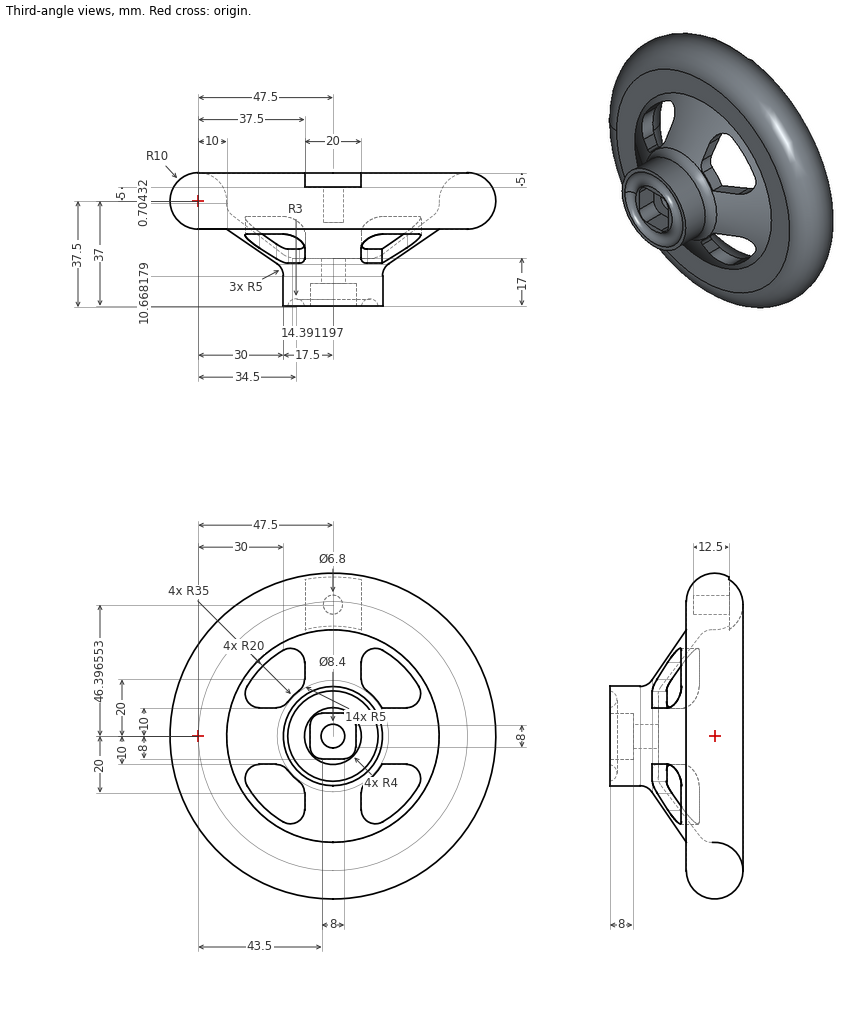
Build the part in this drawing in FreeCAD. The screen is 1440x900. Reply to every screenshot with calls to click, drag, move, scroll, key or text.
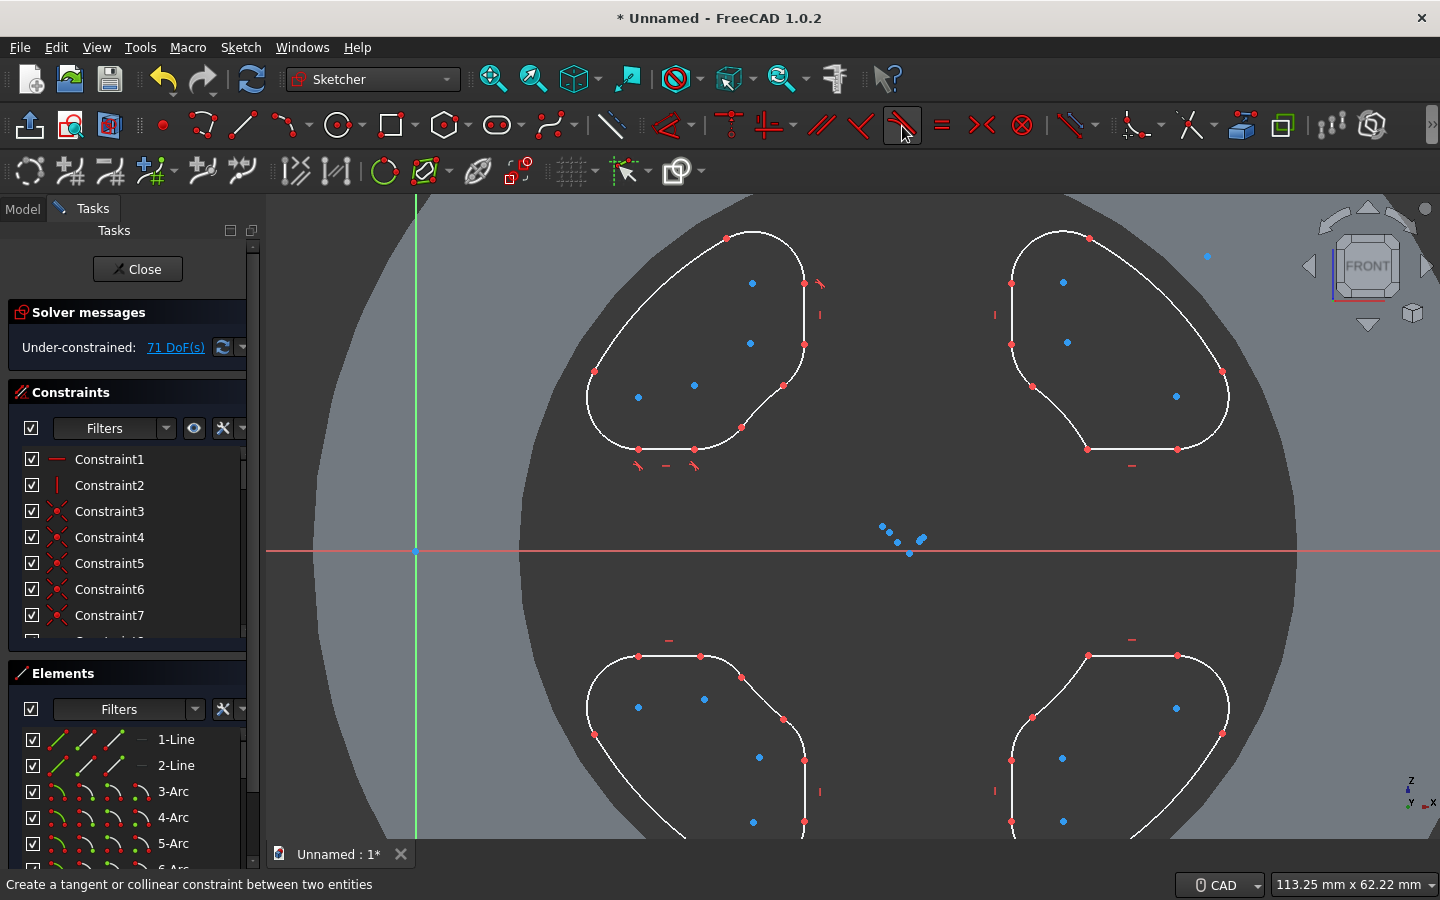
click(804, 302)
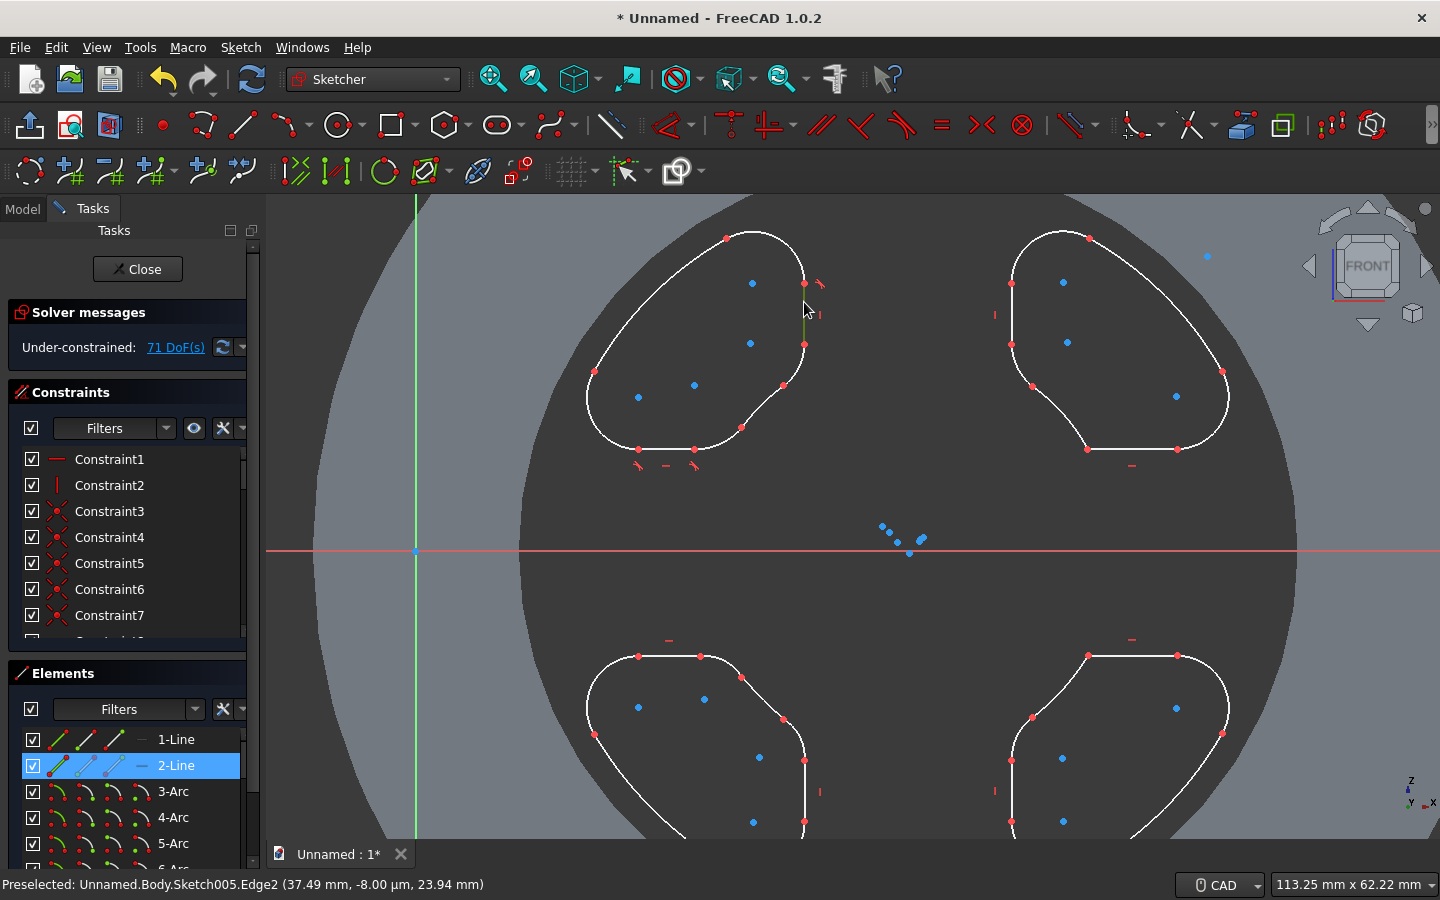
click(794, 376)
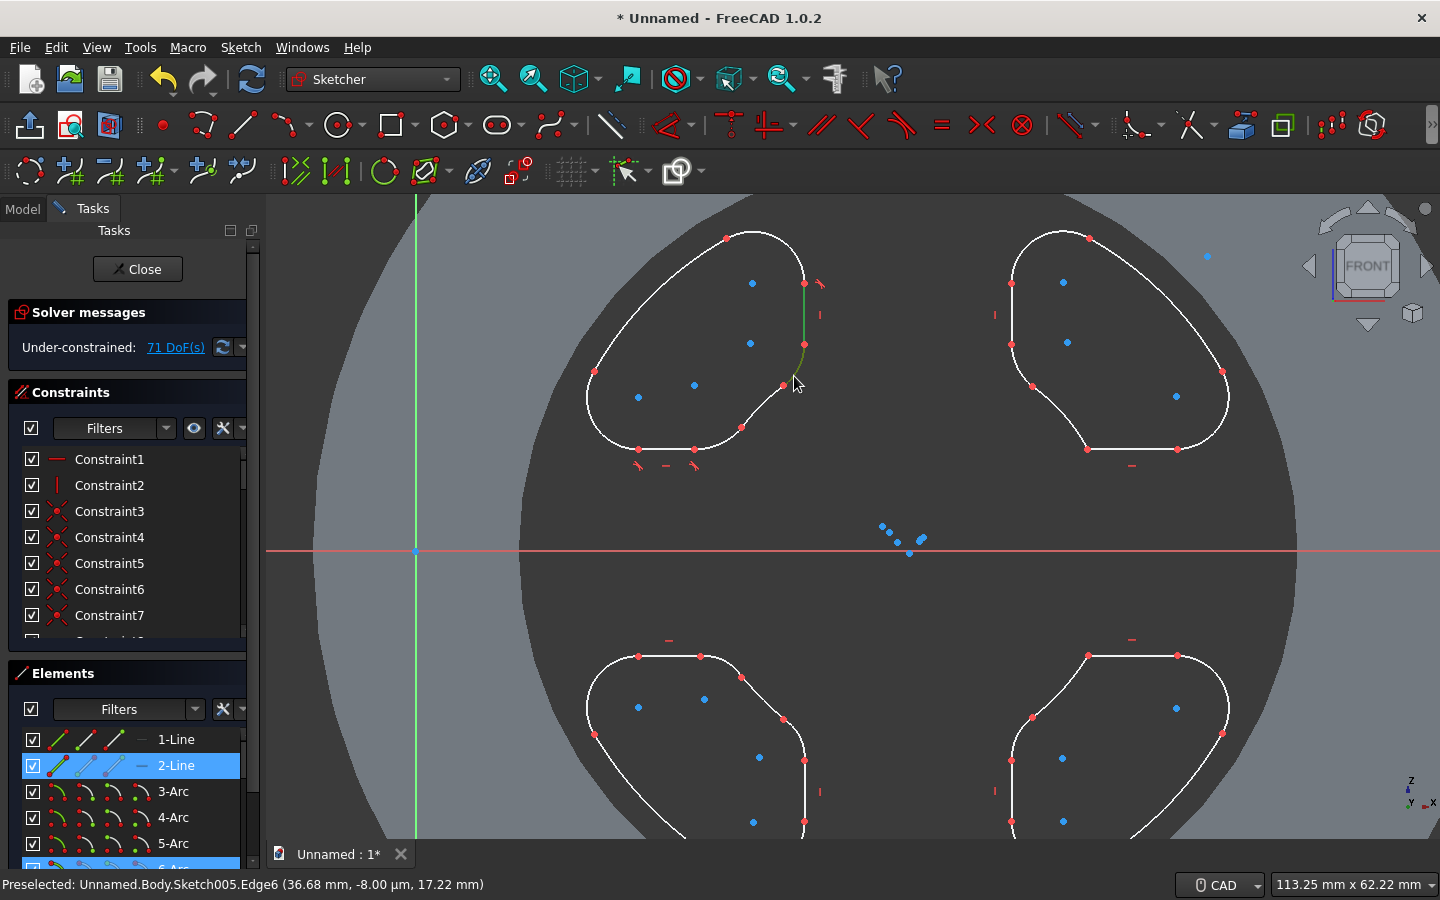
click(902, 126)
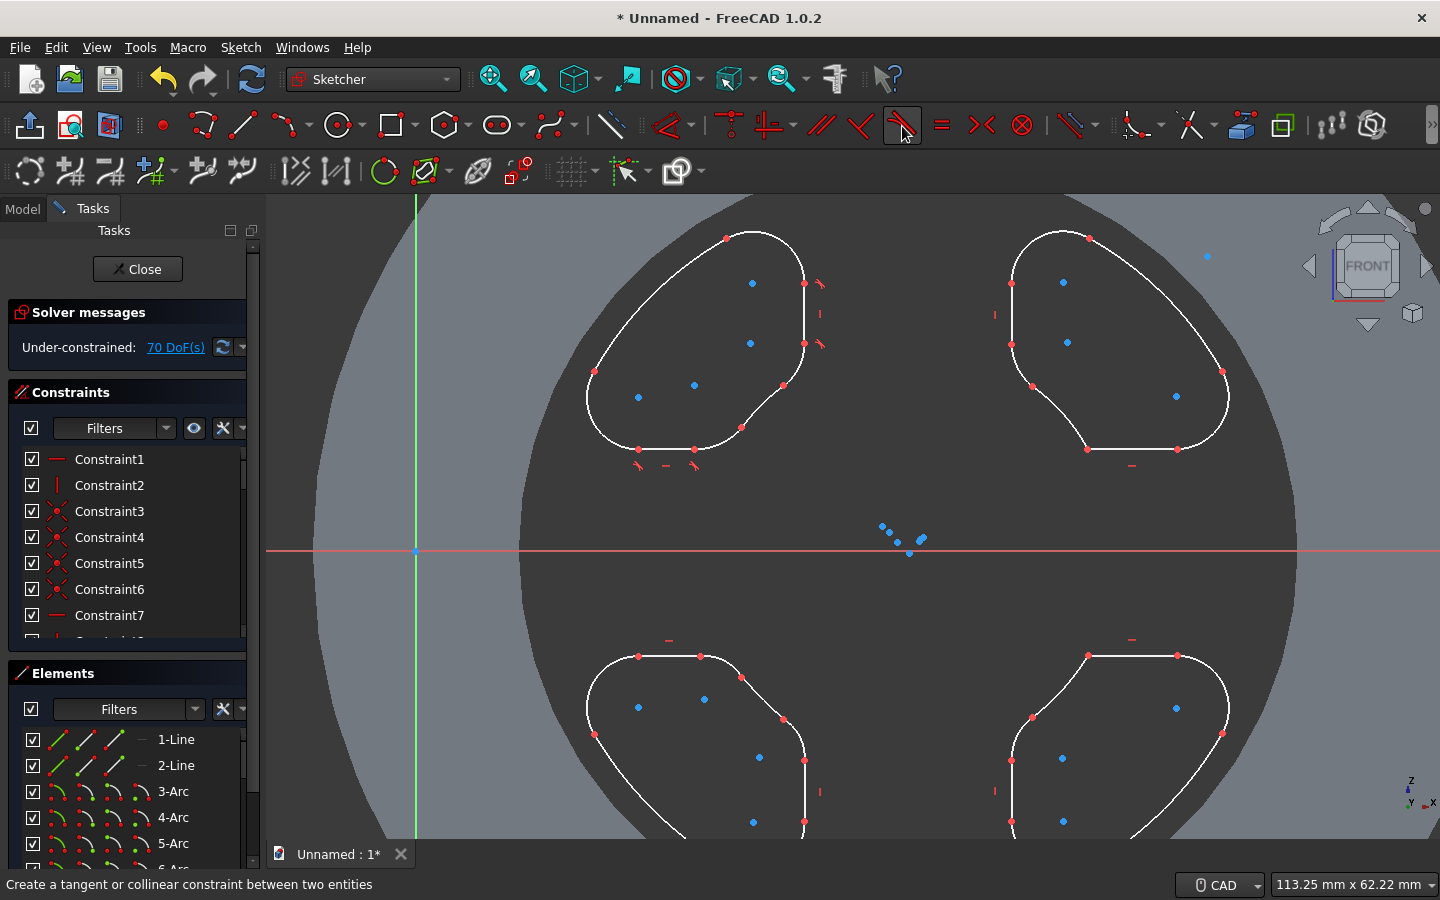
click(587, 403)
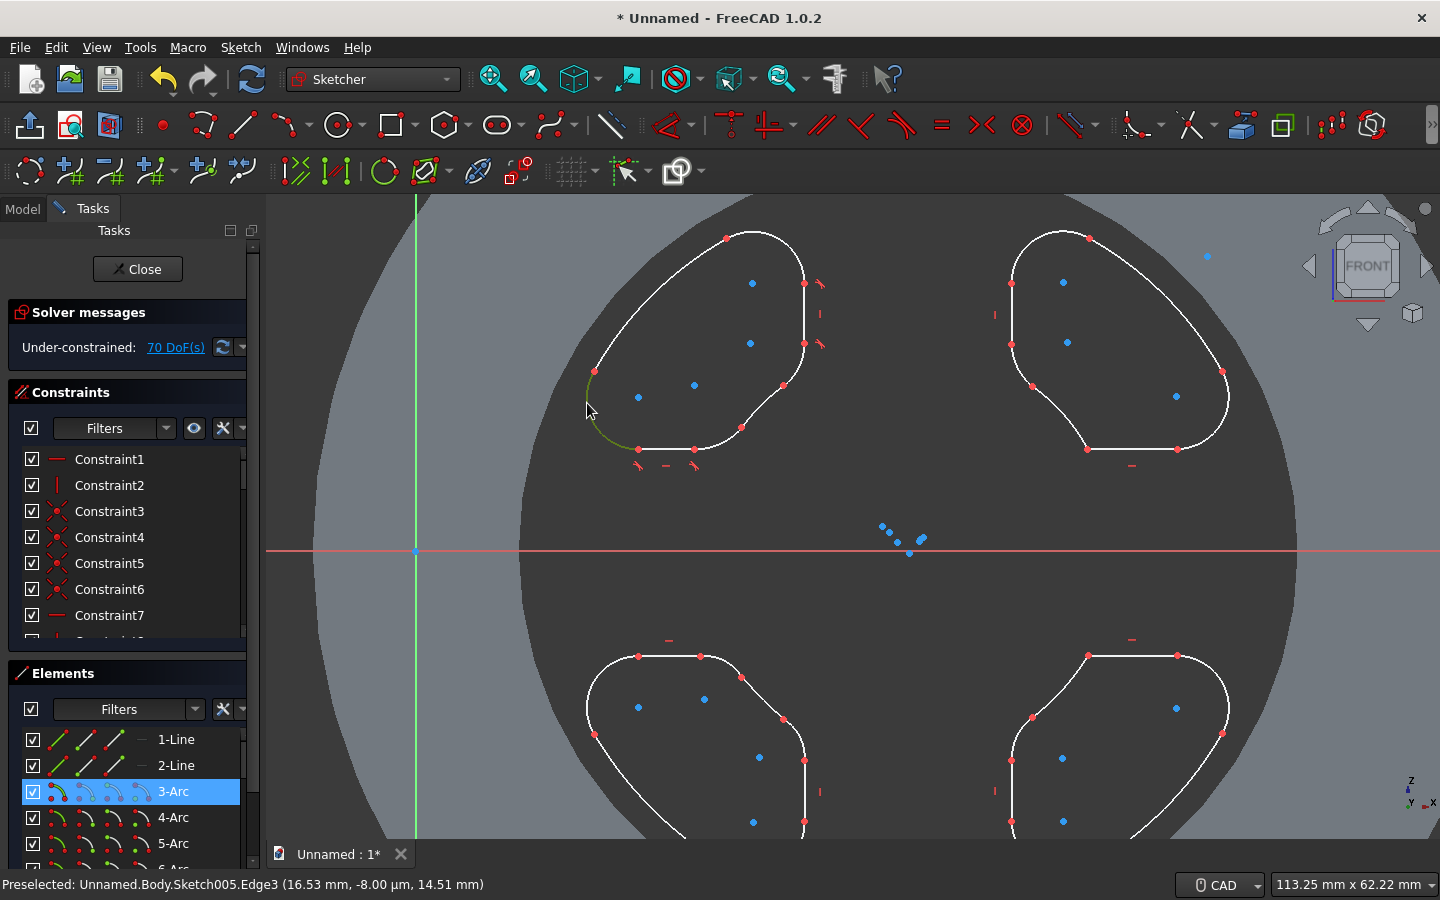
click(680, 271)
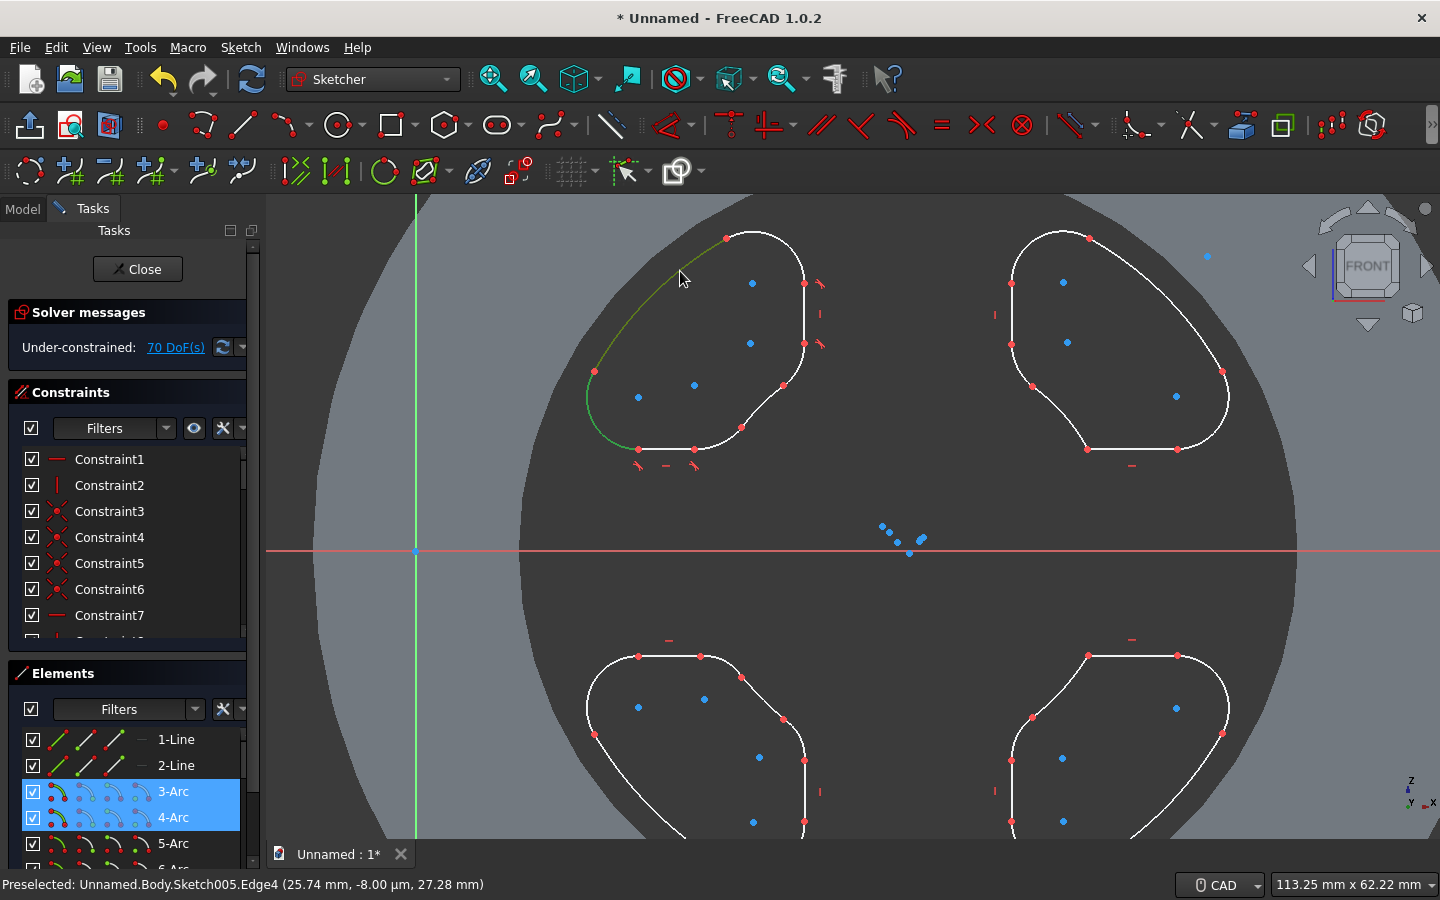
click(902, 126)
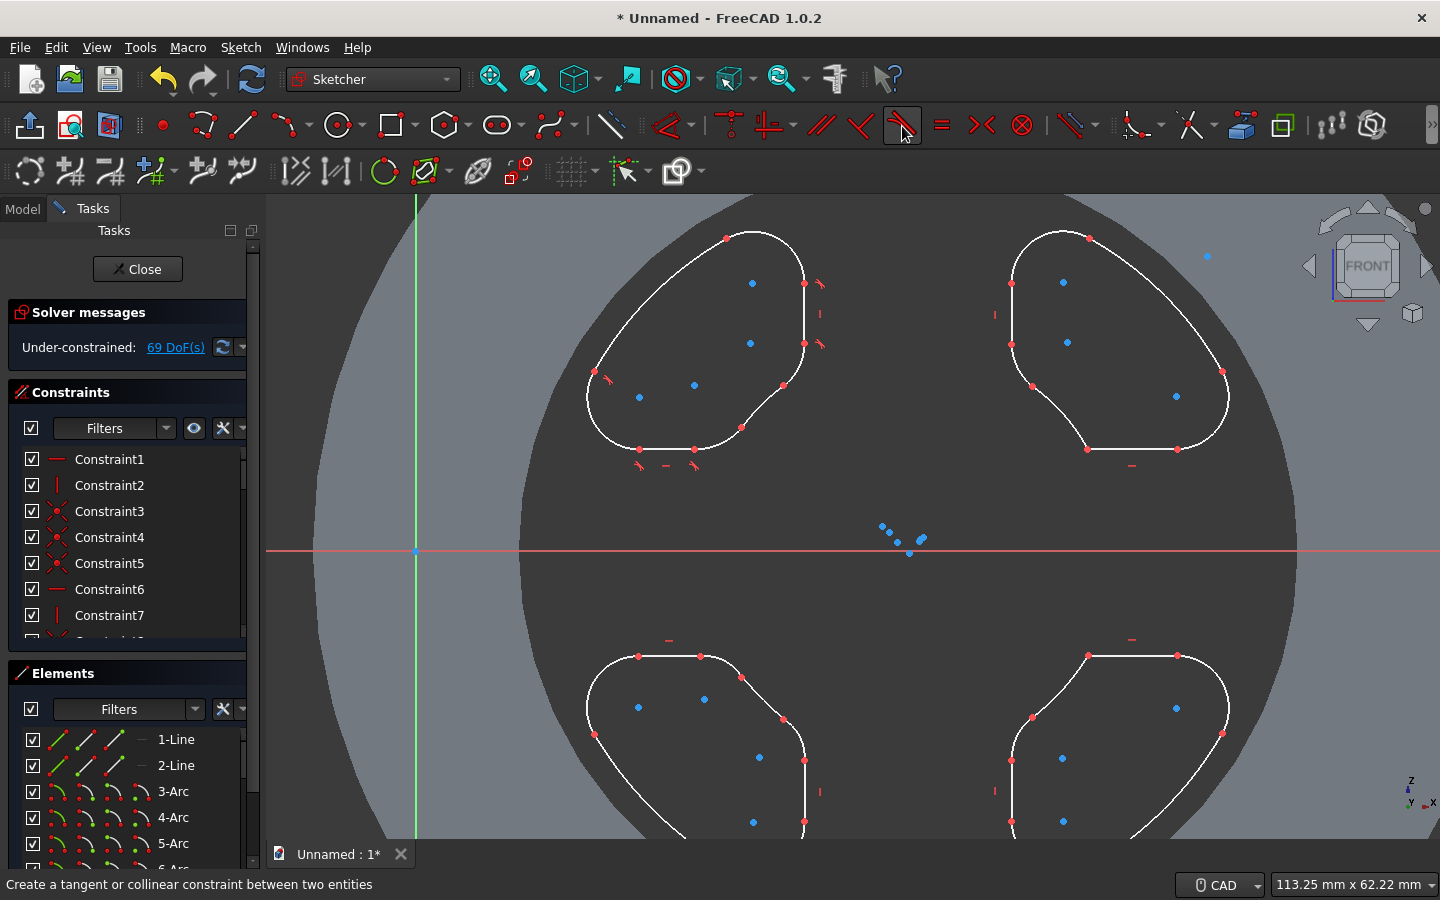
click(680, 271)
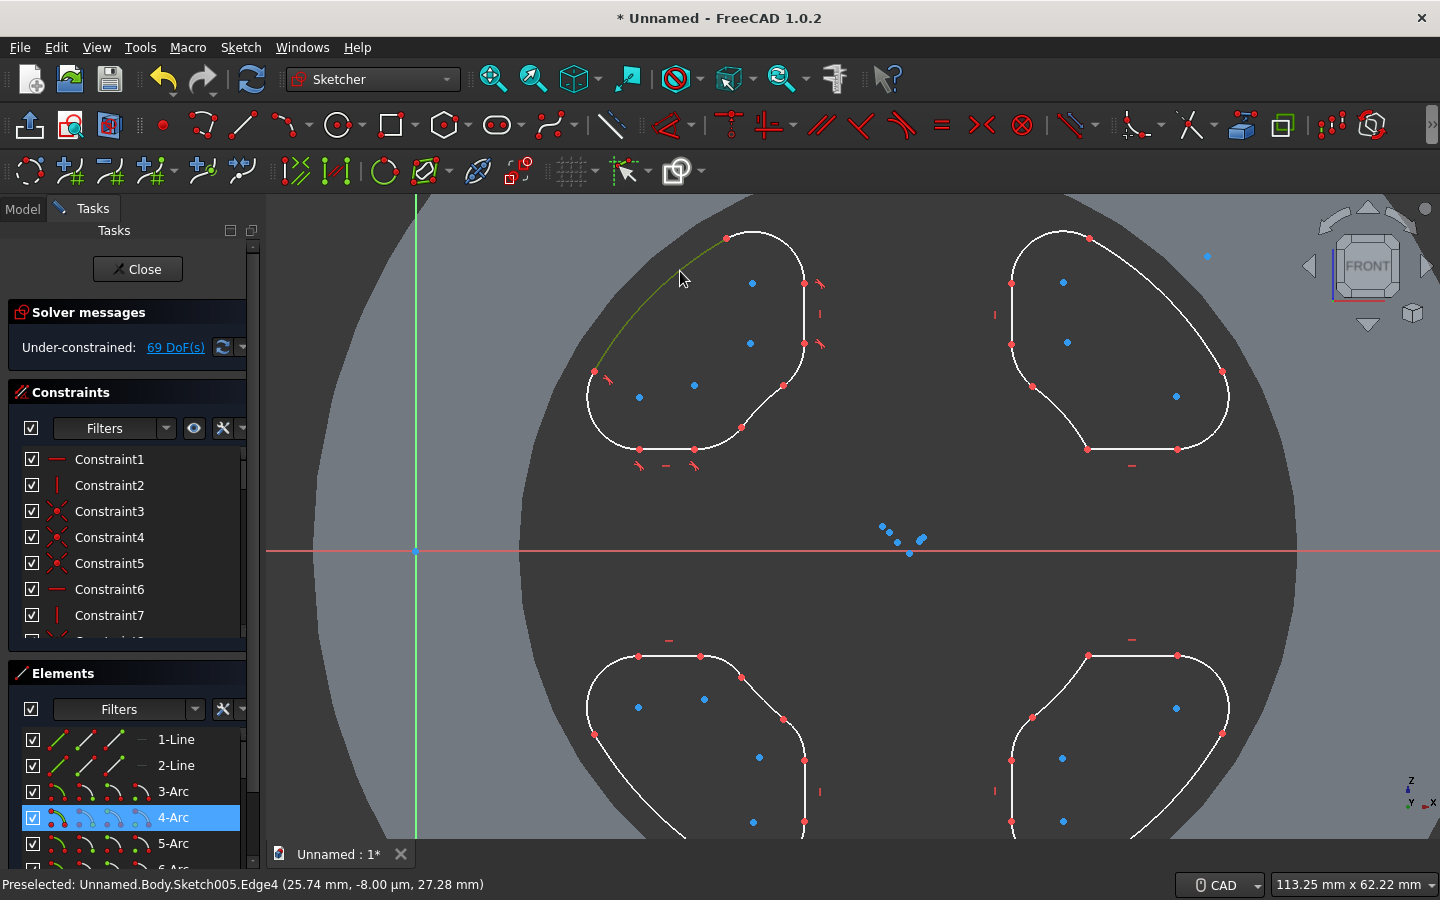
click(795, 253)